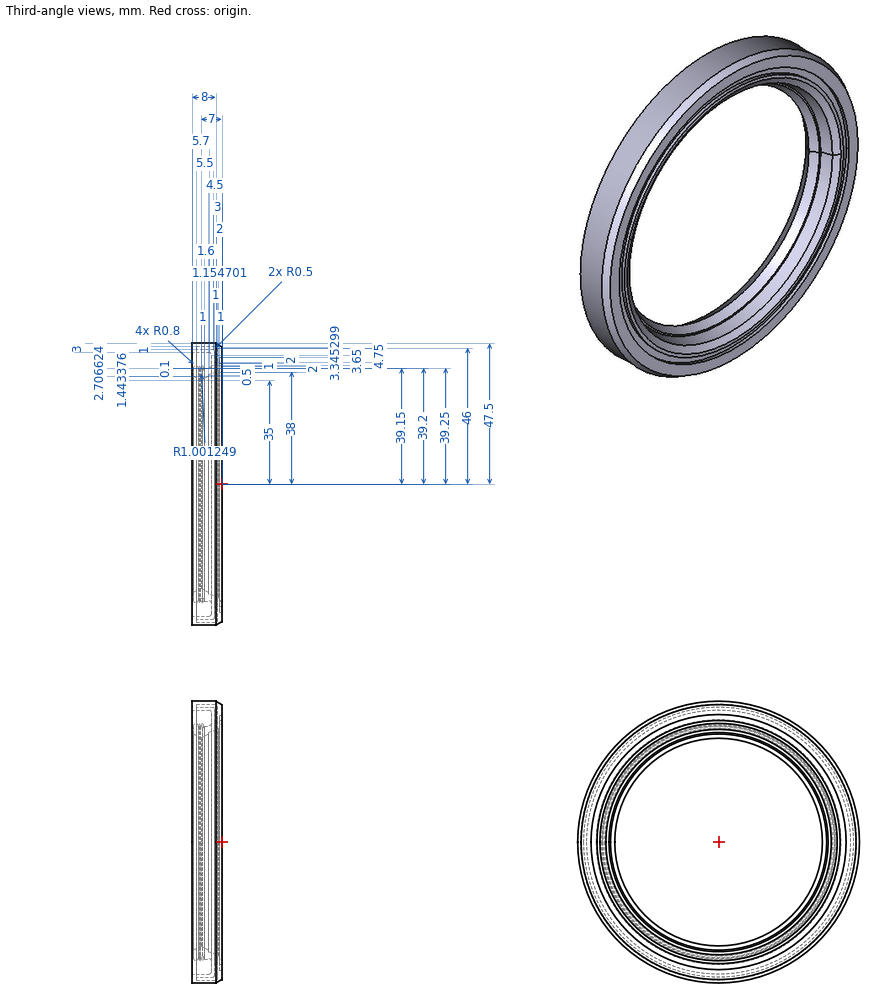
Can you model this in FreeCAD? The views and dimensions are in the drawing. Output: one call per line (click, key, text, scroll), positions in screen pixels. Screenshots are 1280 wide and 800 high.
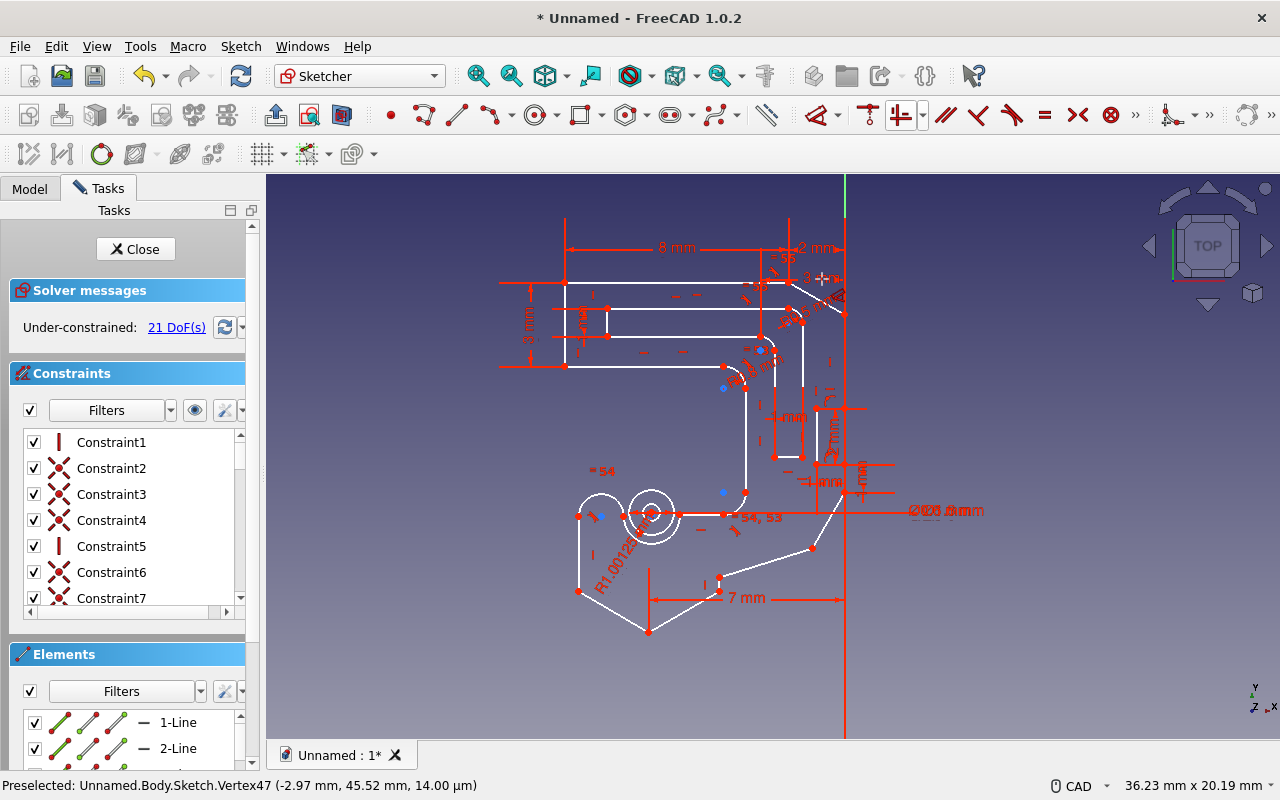
click(822, 532)
click(879, 521)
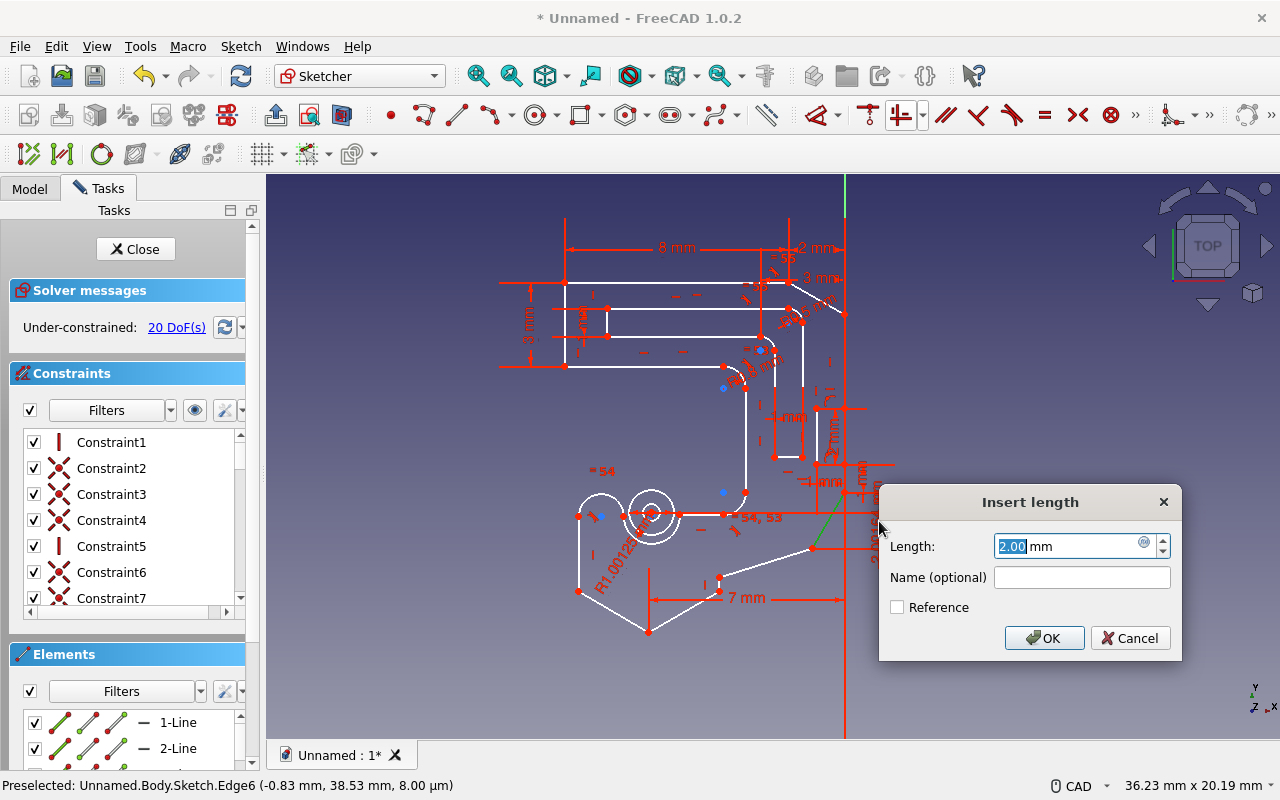
text(2)
key(Return)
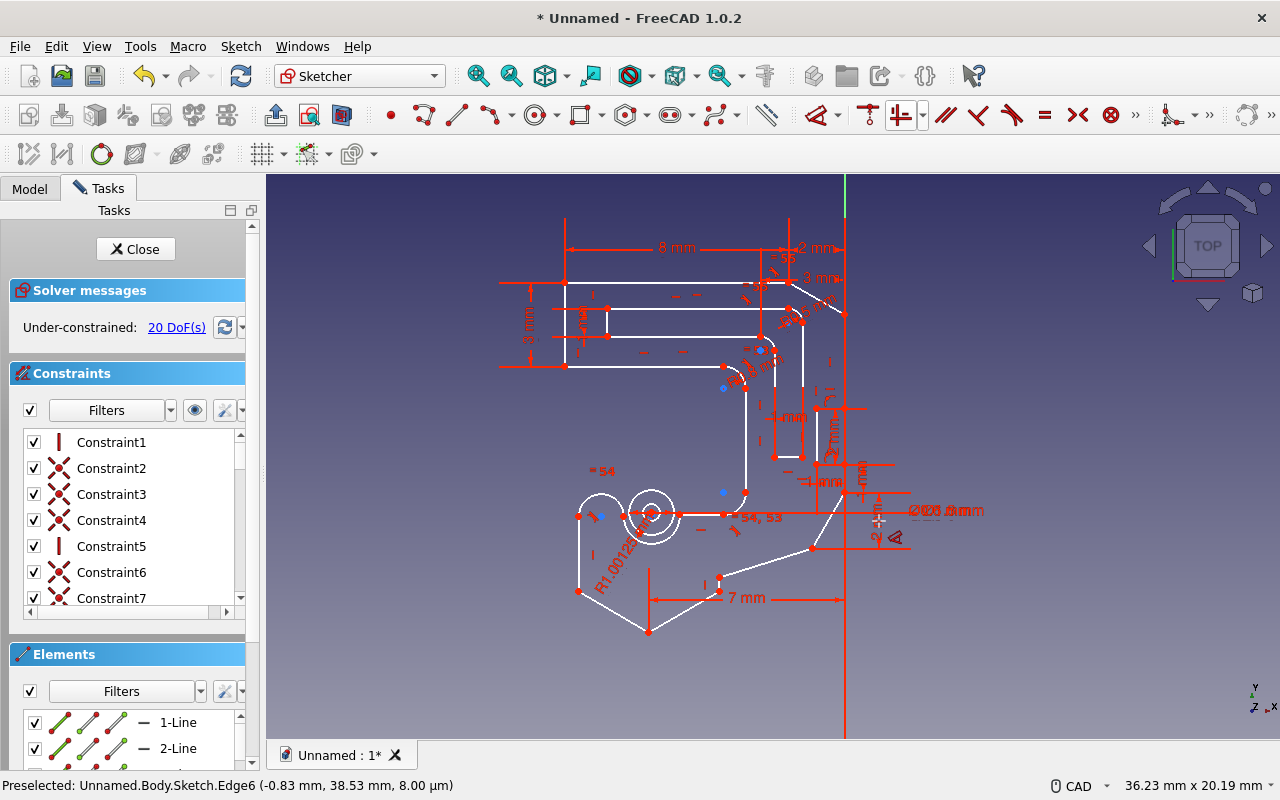
scroll(680, 515, up, 2)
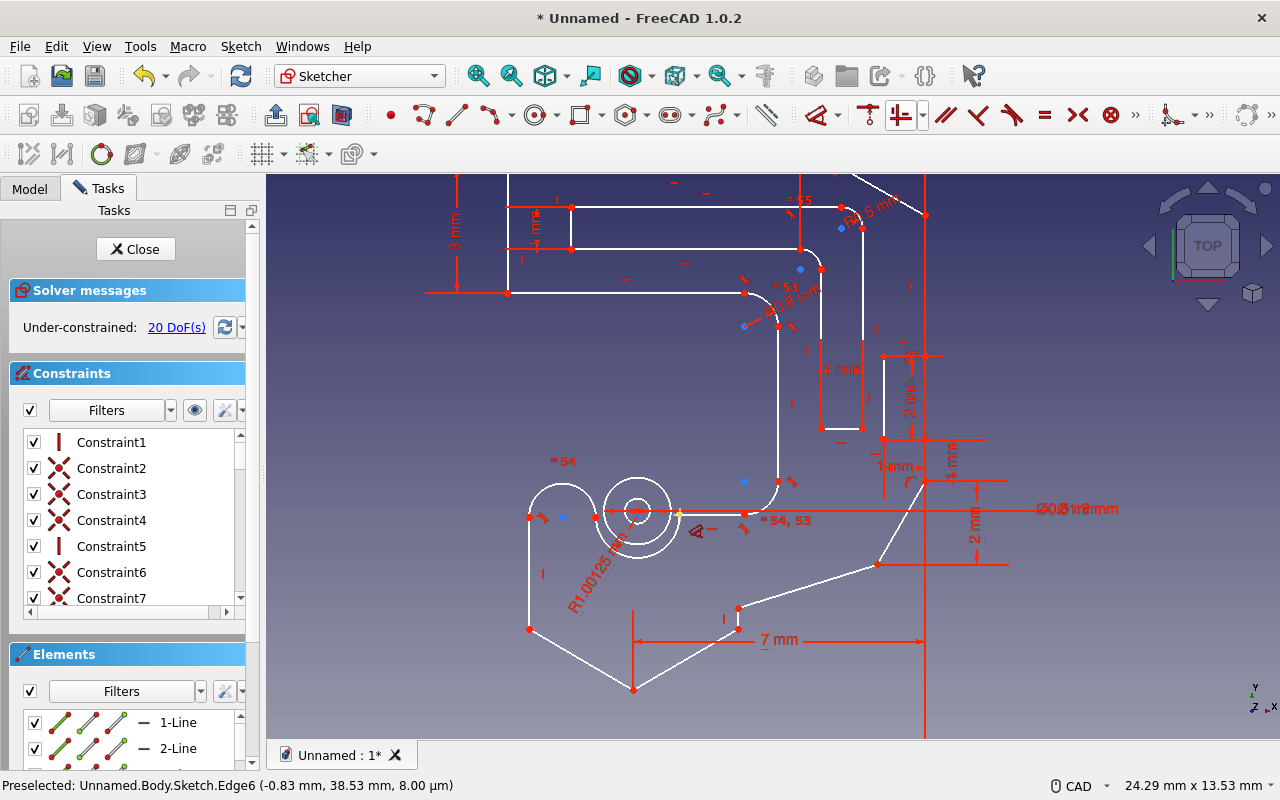
click(679, 515)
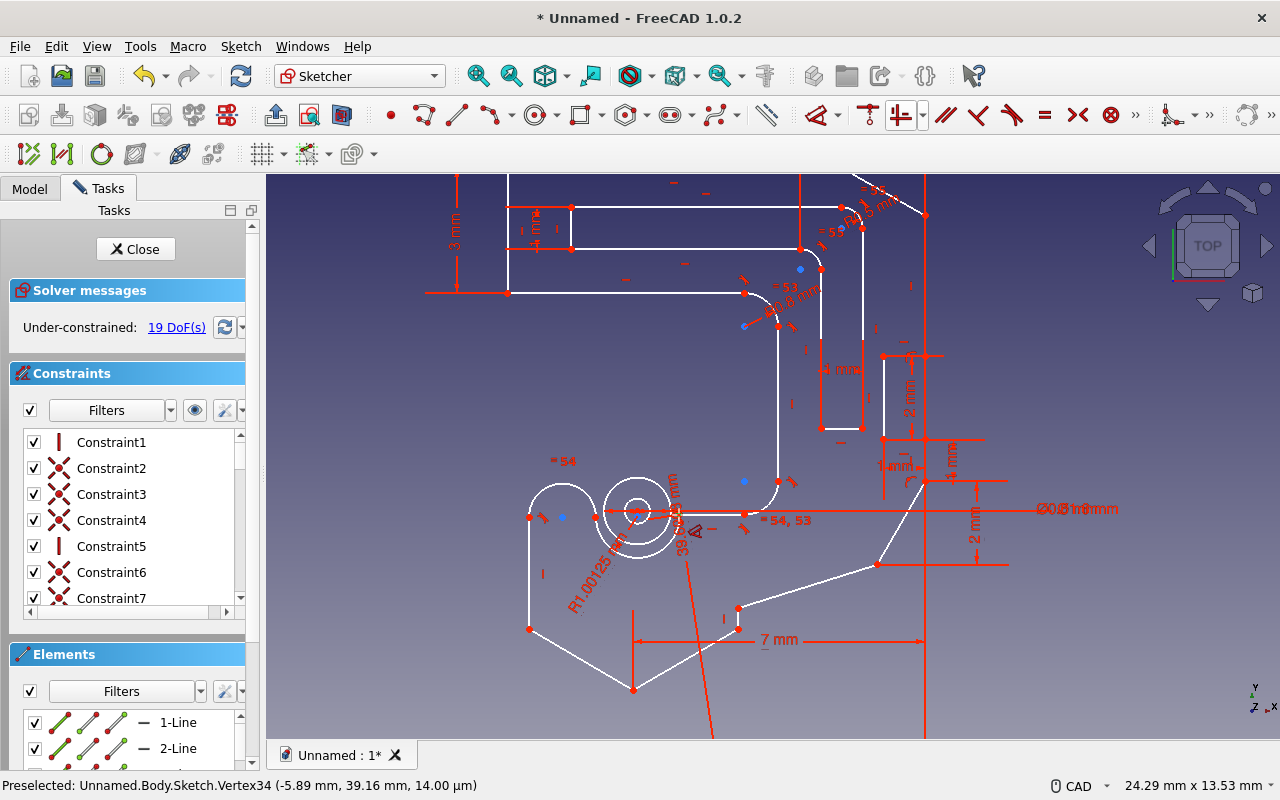
scroll(637, 511, up, 5)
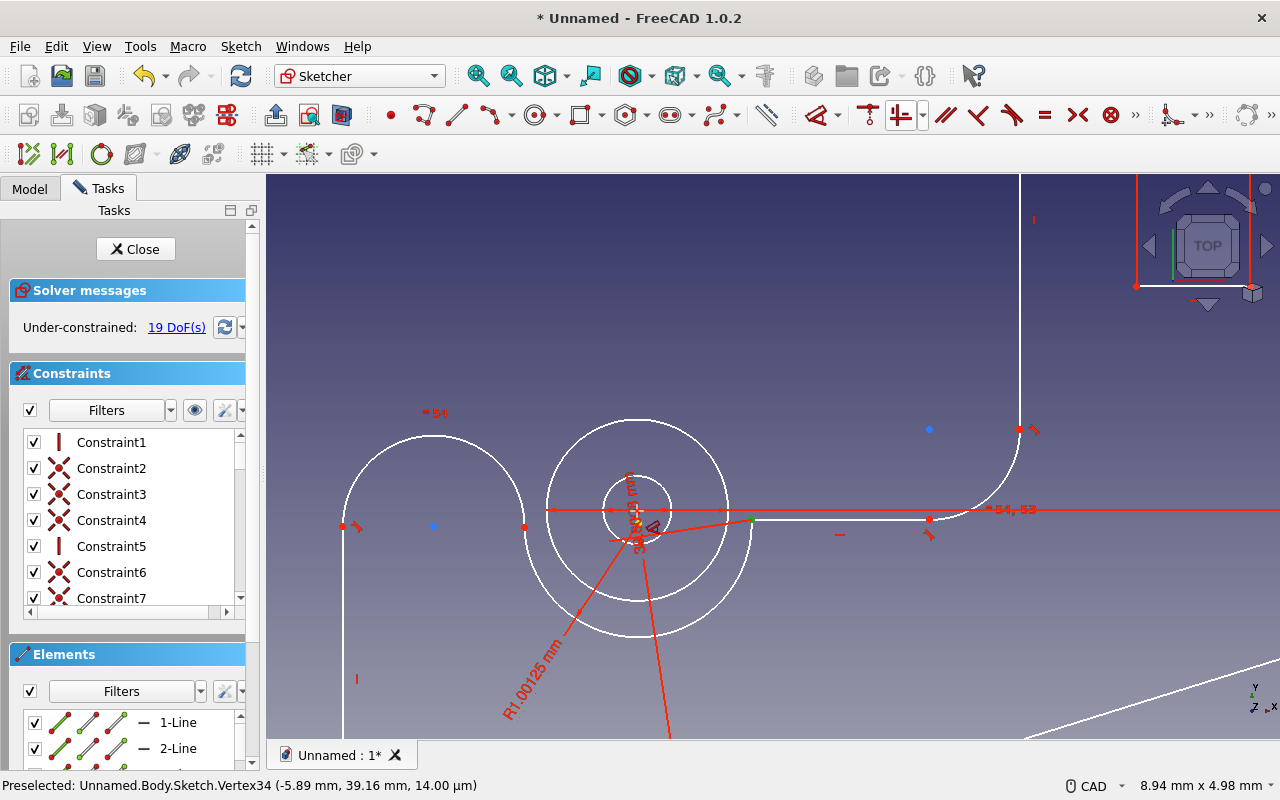
click(637, 510)
click(695, 554)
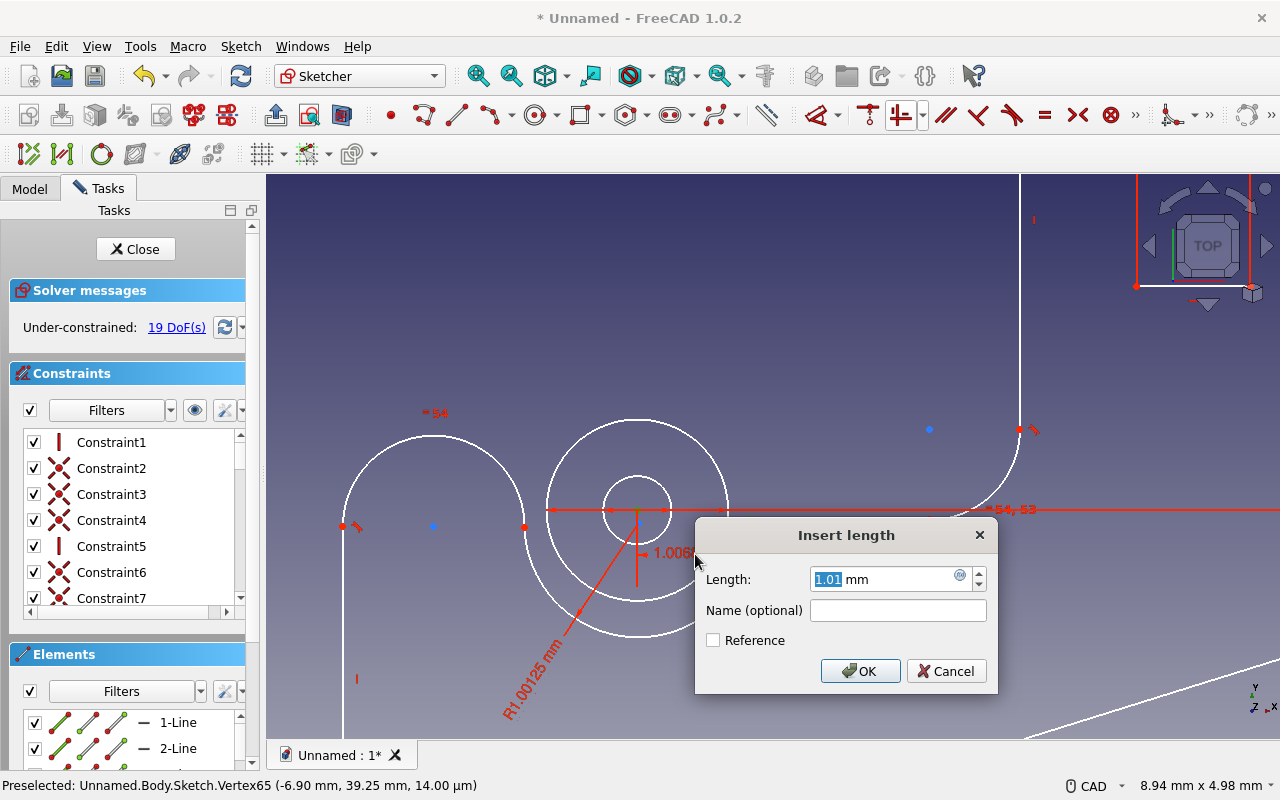
text(1)
key(Return)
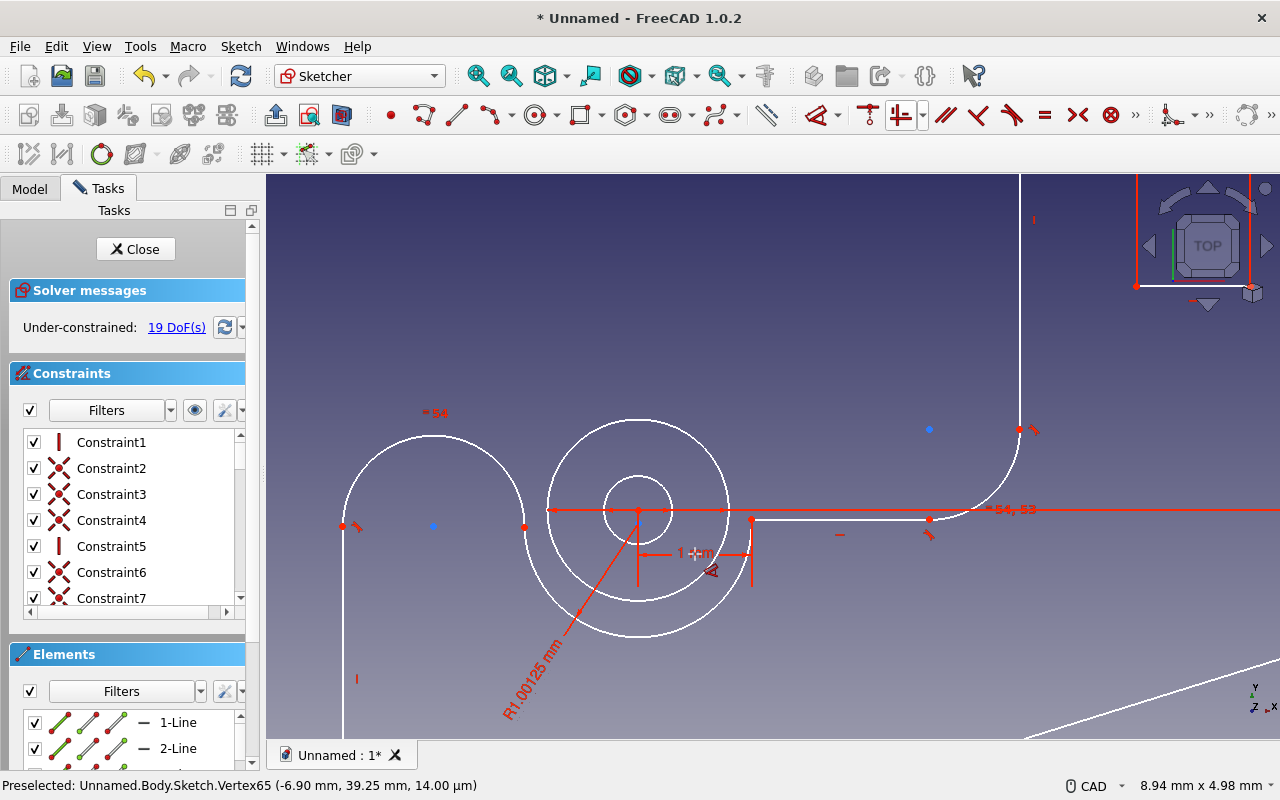
scroll(656, 513, down, 7)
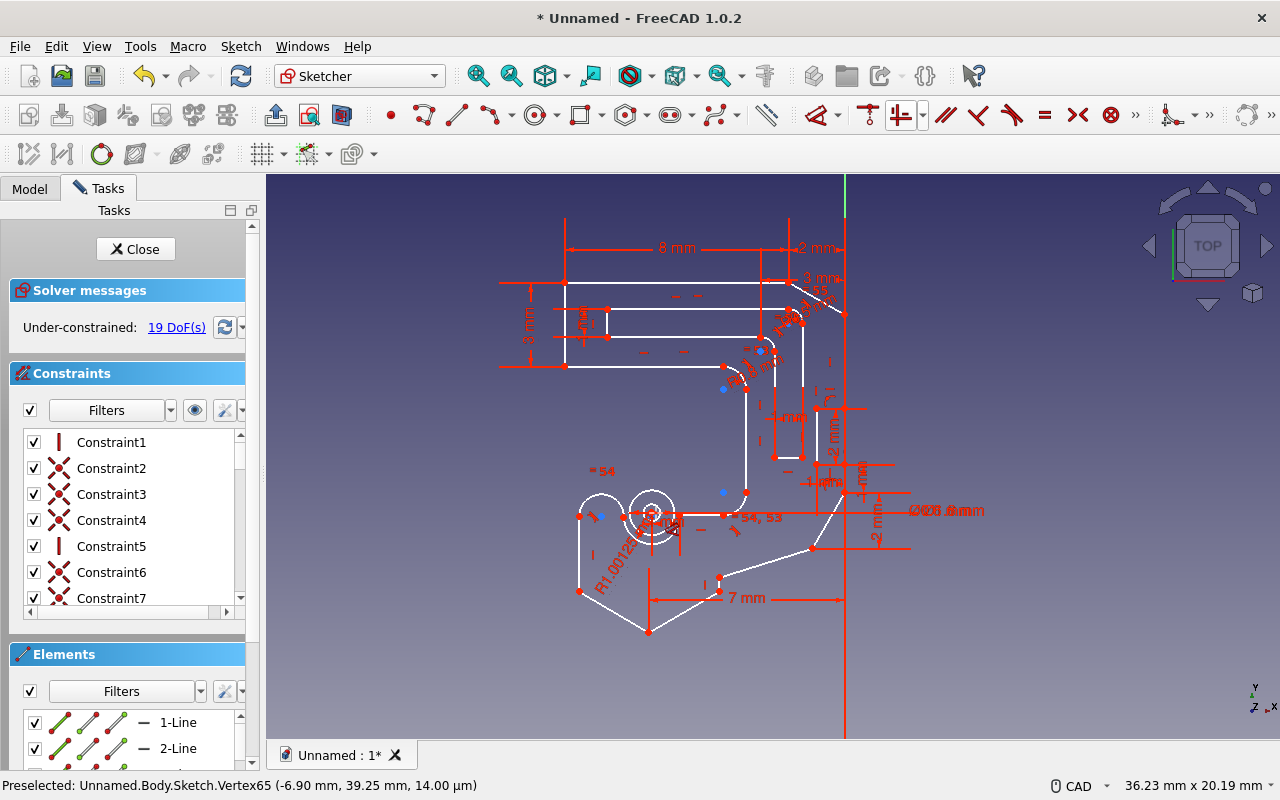
scroll(719, 588, up, 6)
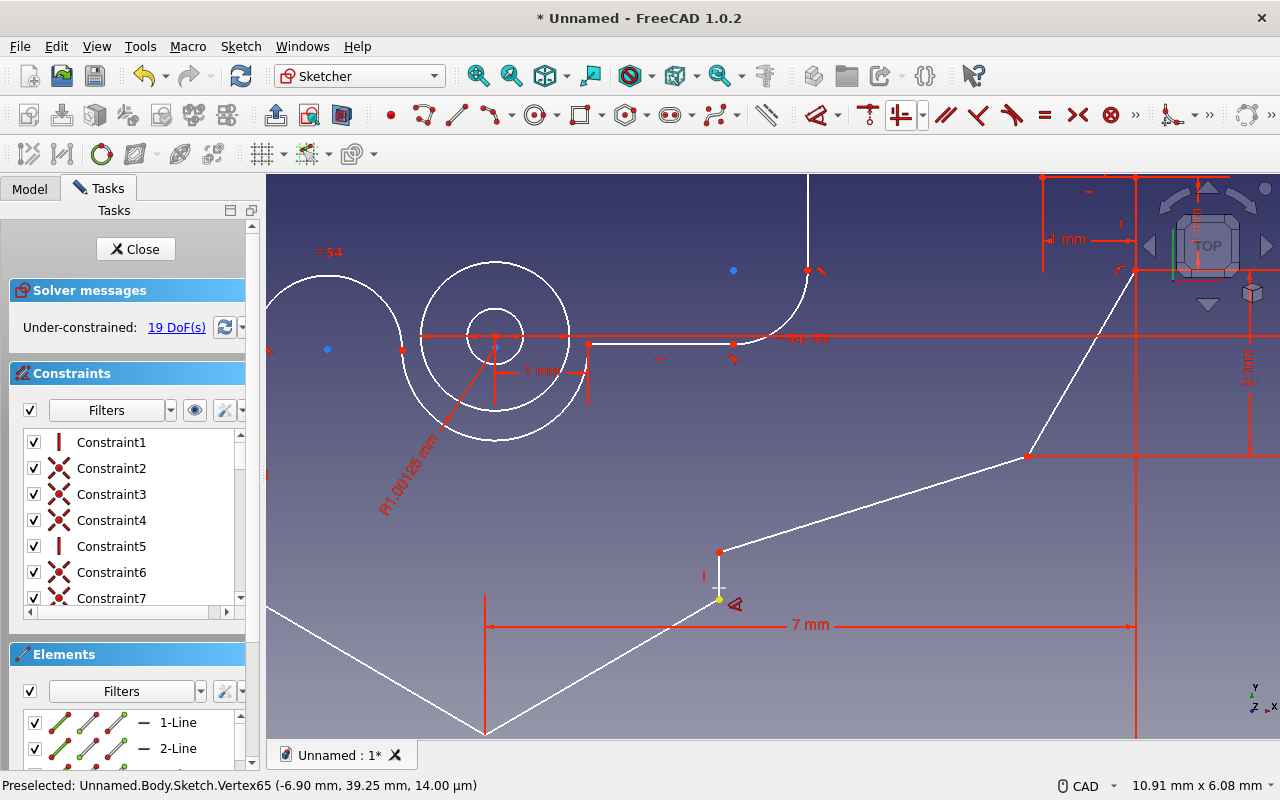
click(719, 585)
click(753, 576)